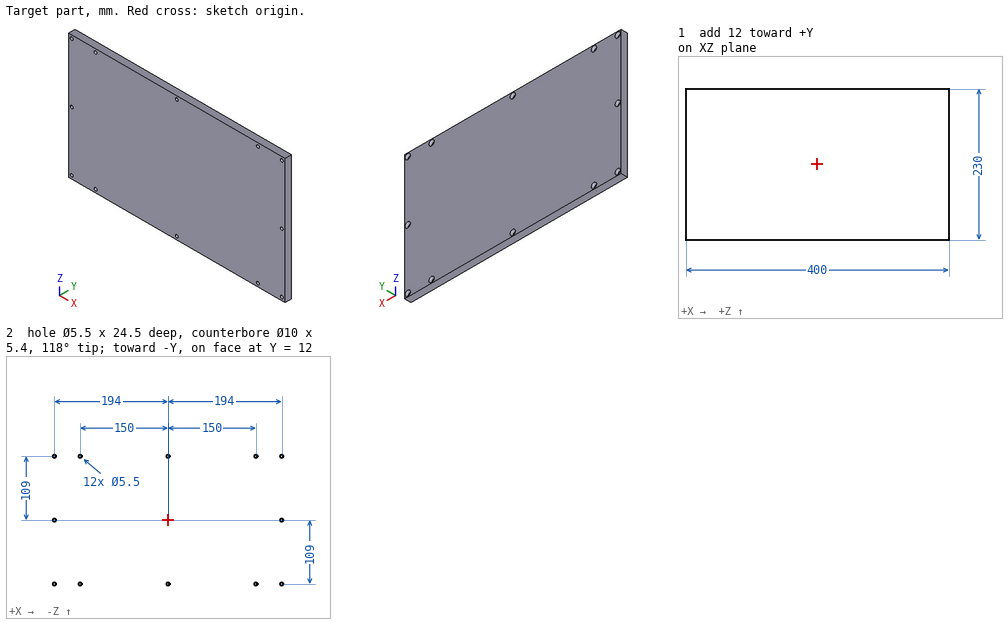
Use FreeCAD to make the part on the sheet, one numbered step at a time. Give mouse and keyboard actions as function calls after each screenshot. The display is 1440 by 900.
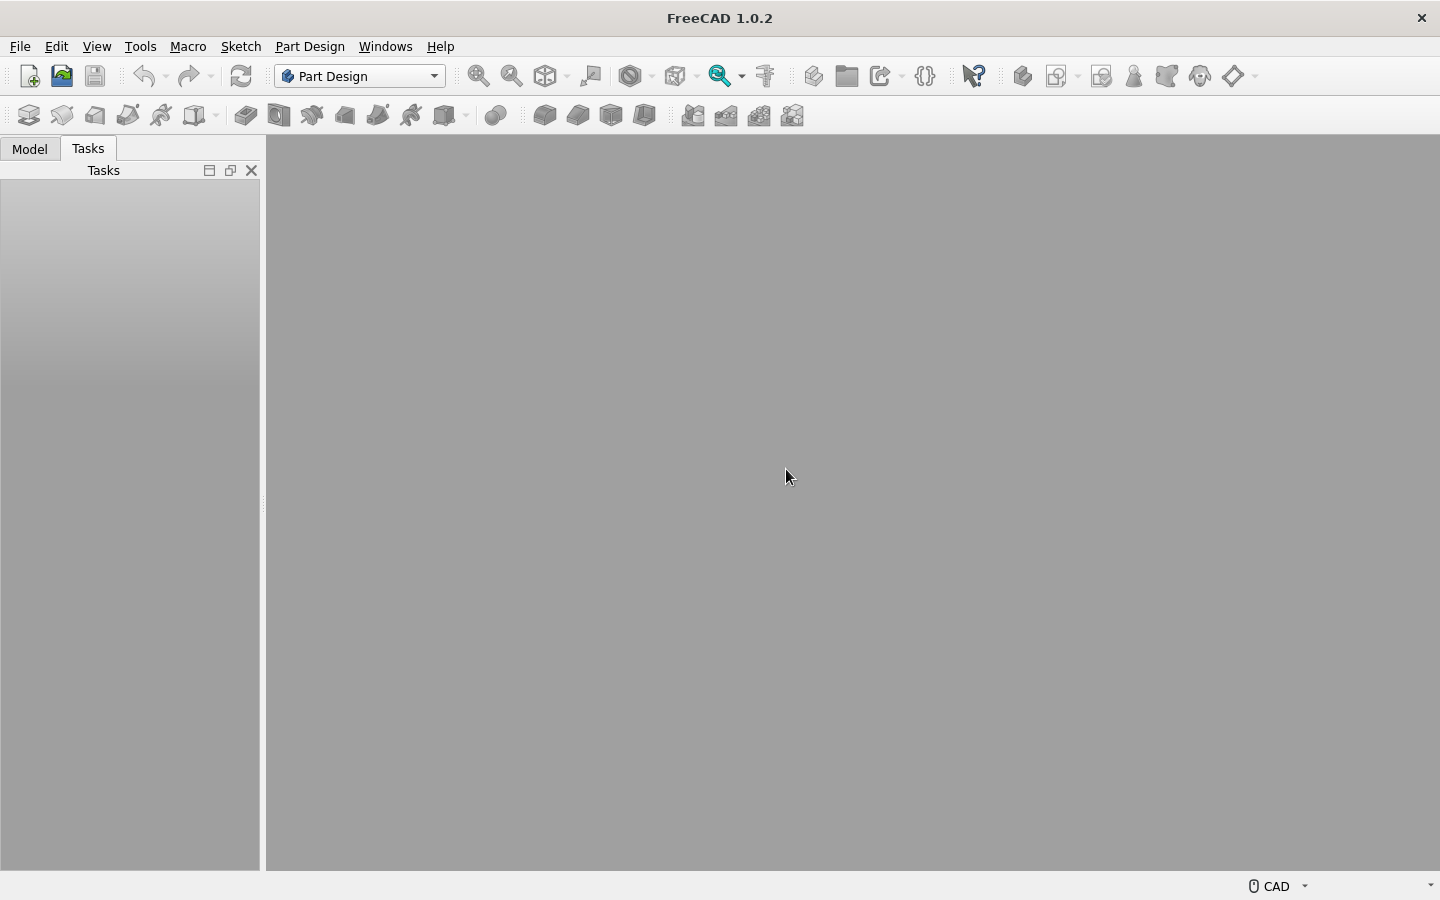
click(29, 76)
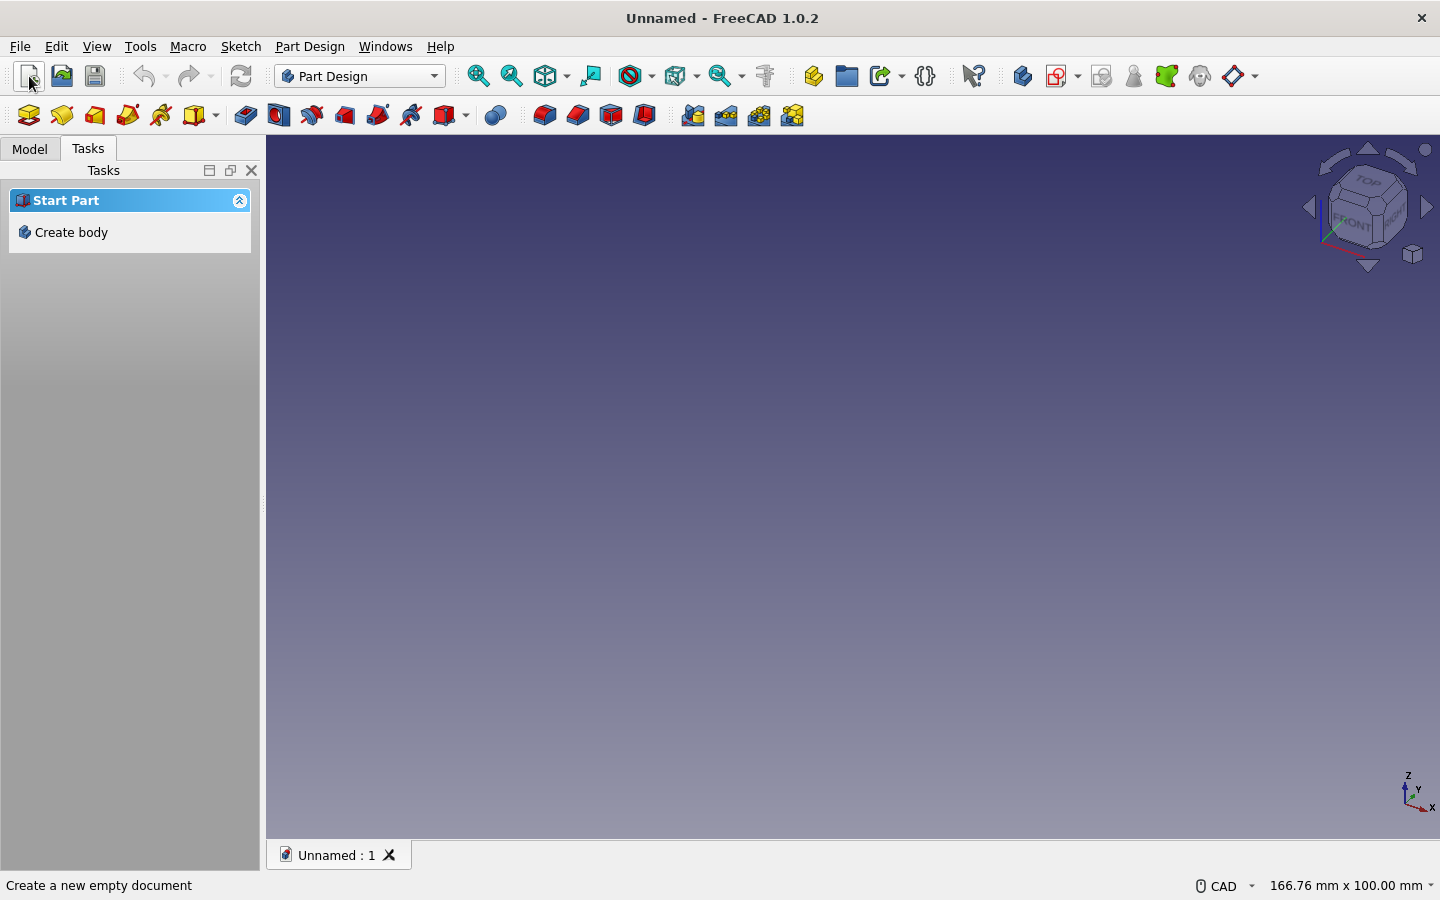
click(1056, 76)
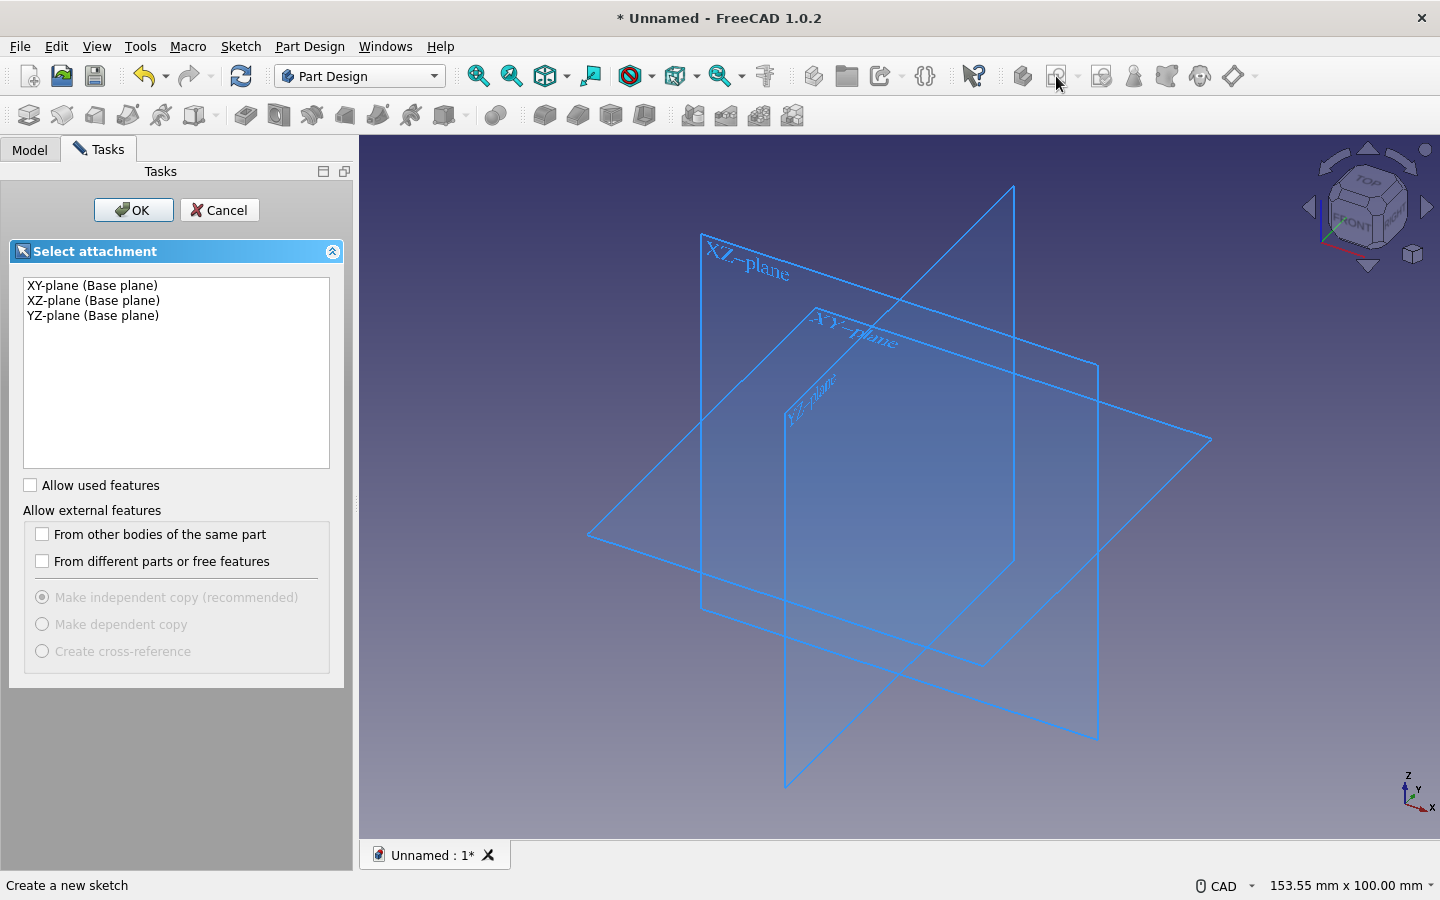
click(84, 300)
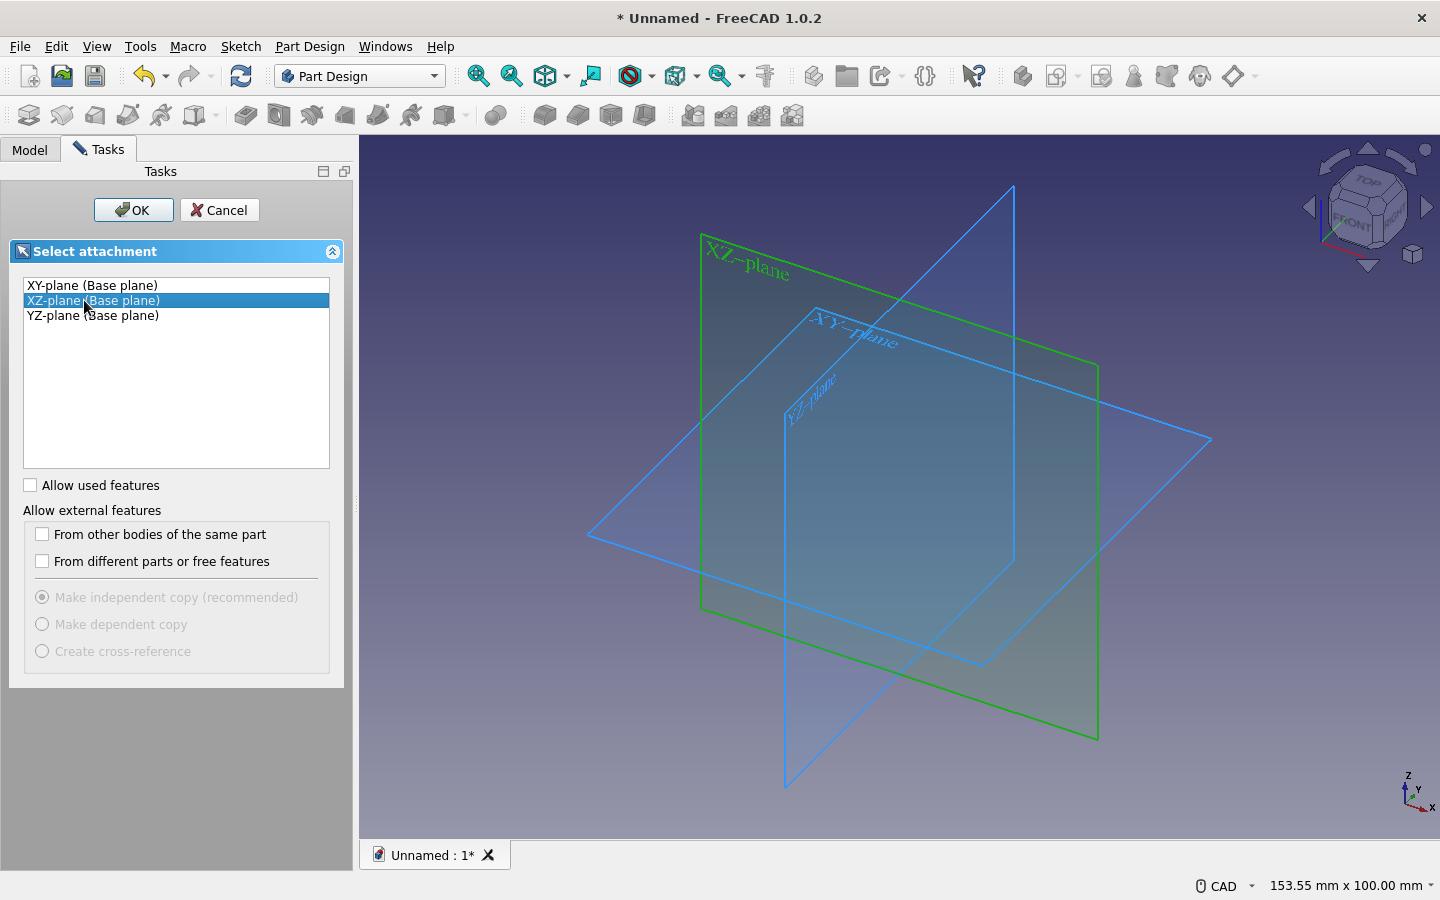
click(134, 210)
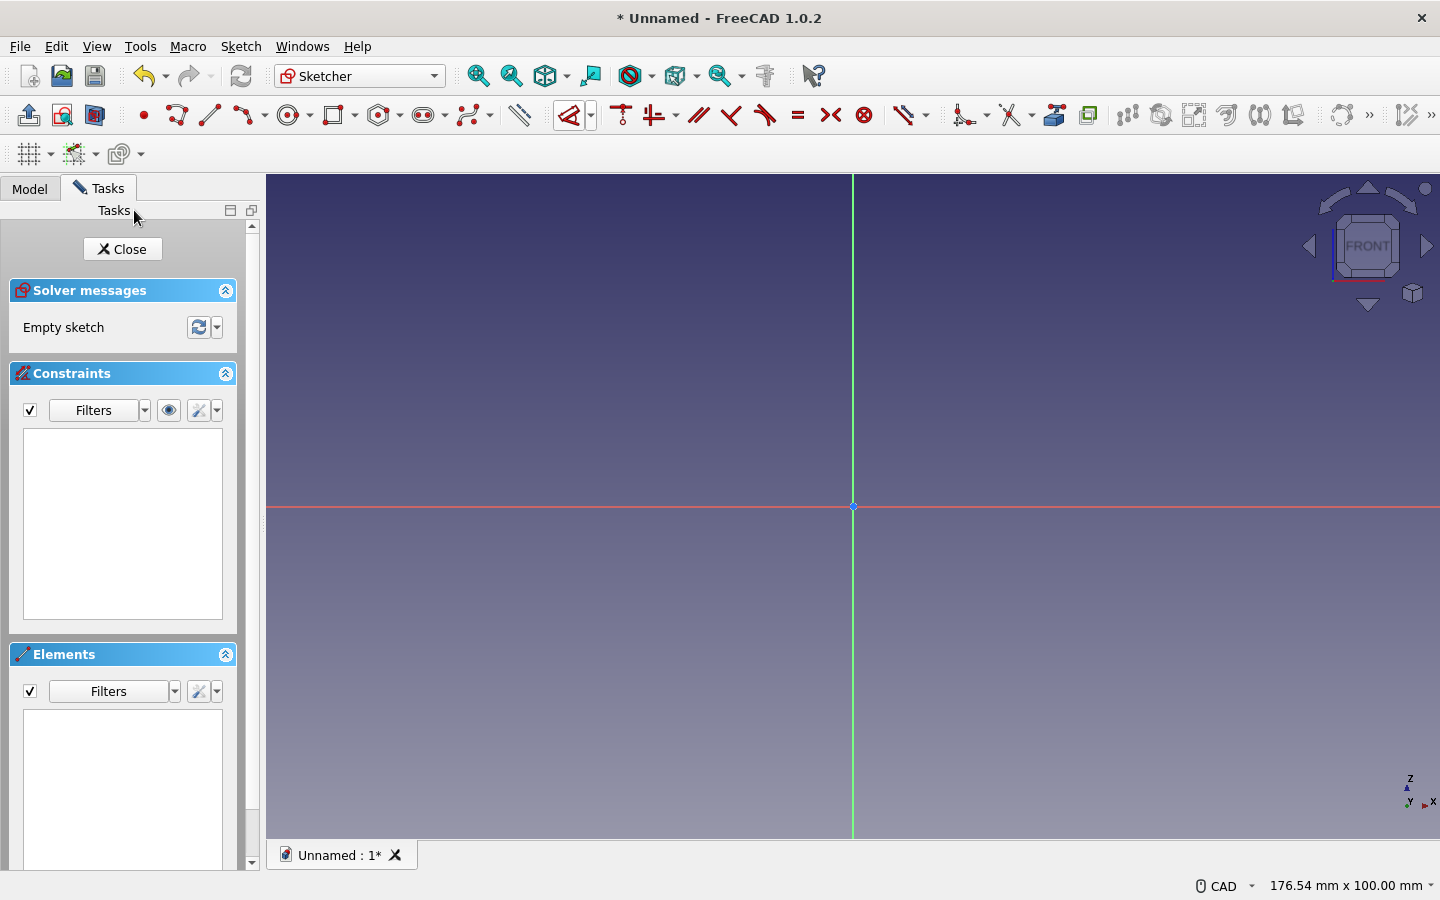
scroll(762, 506, down, 7)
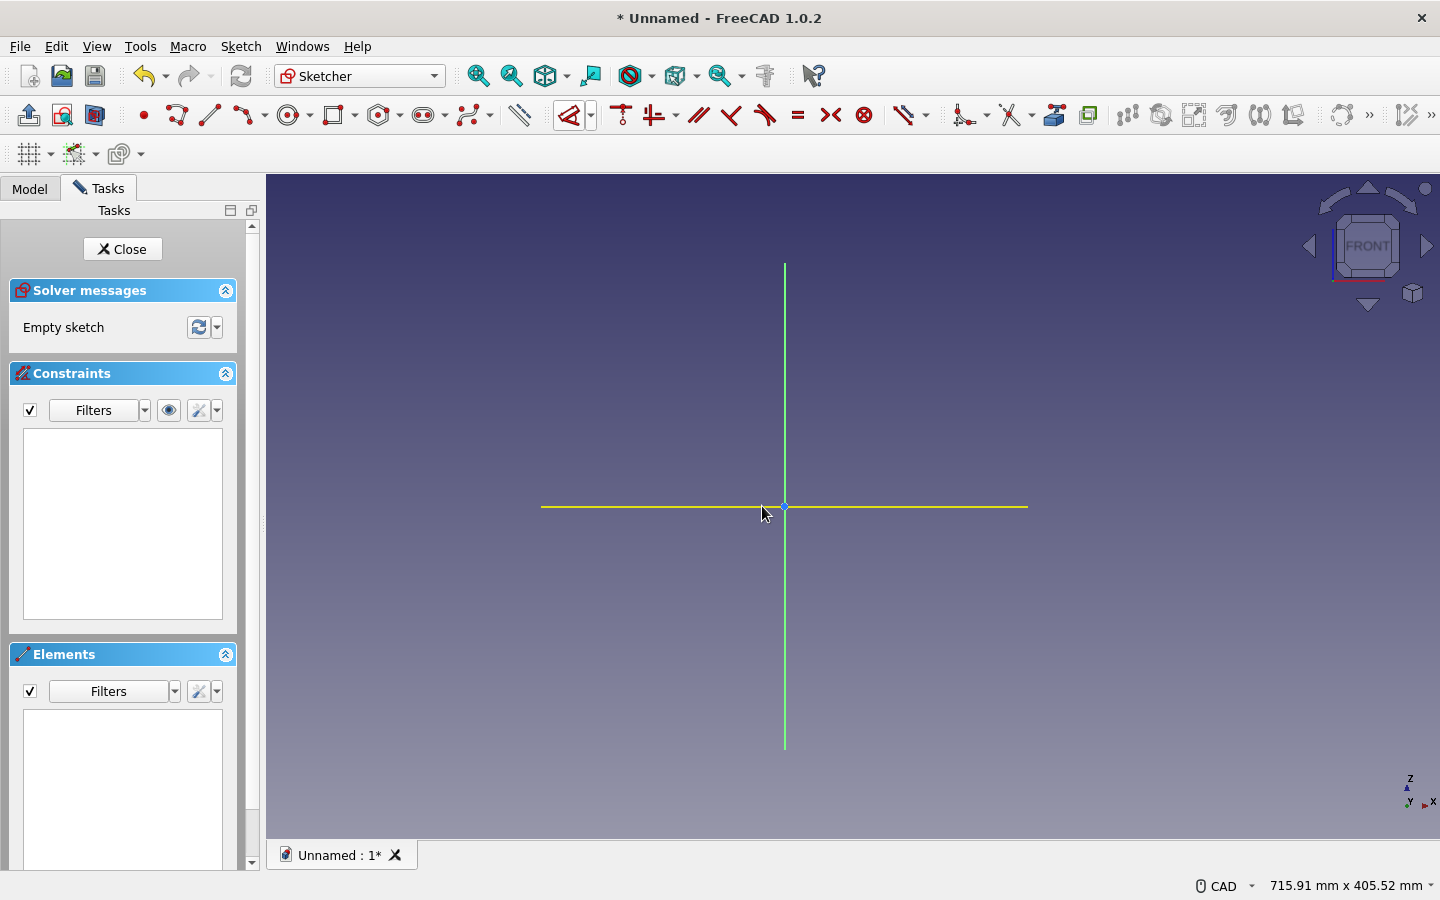
click(354, 116)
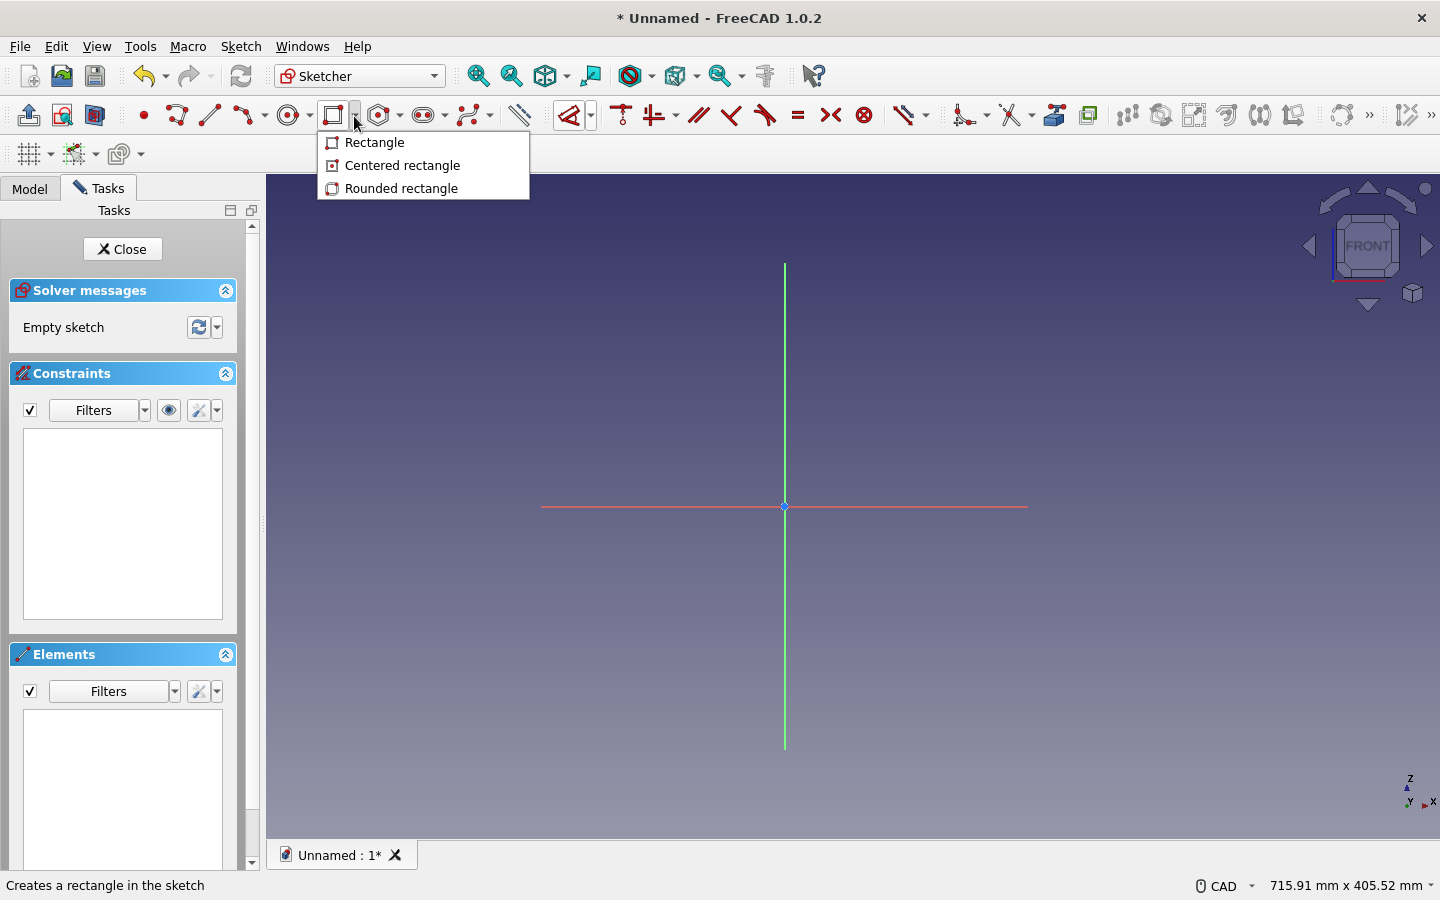
click(424, 166)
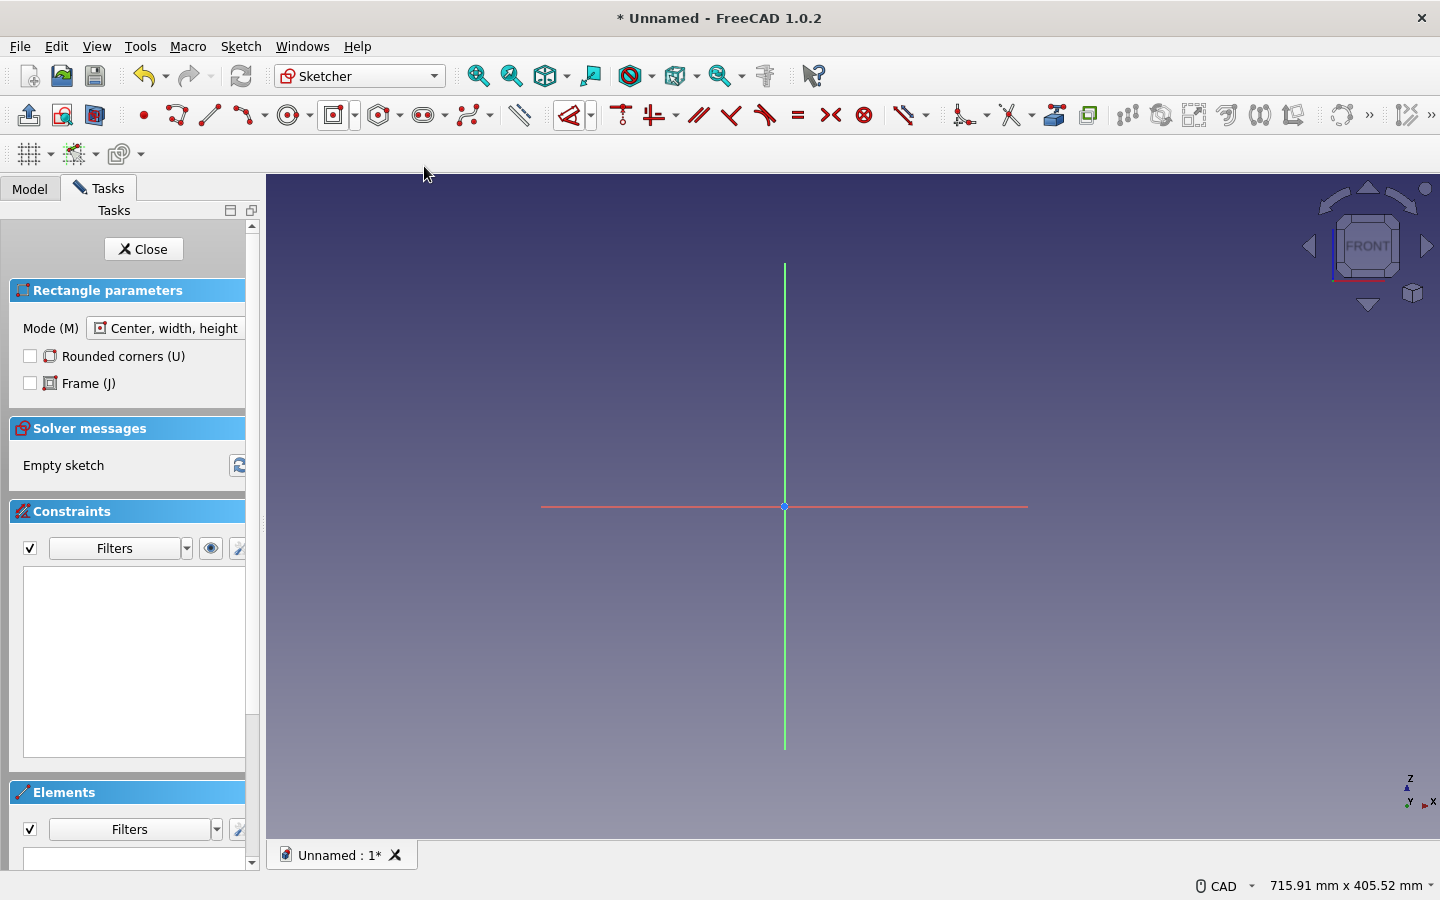
click(785, 506)
move(1113, 318)